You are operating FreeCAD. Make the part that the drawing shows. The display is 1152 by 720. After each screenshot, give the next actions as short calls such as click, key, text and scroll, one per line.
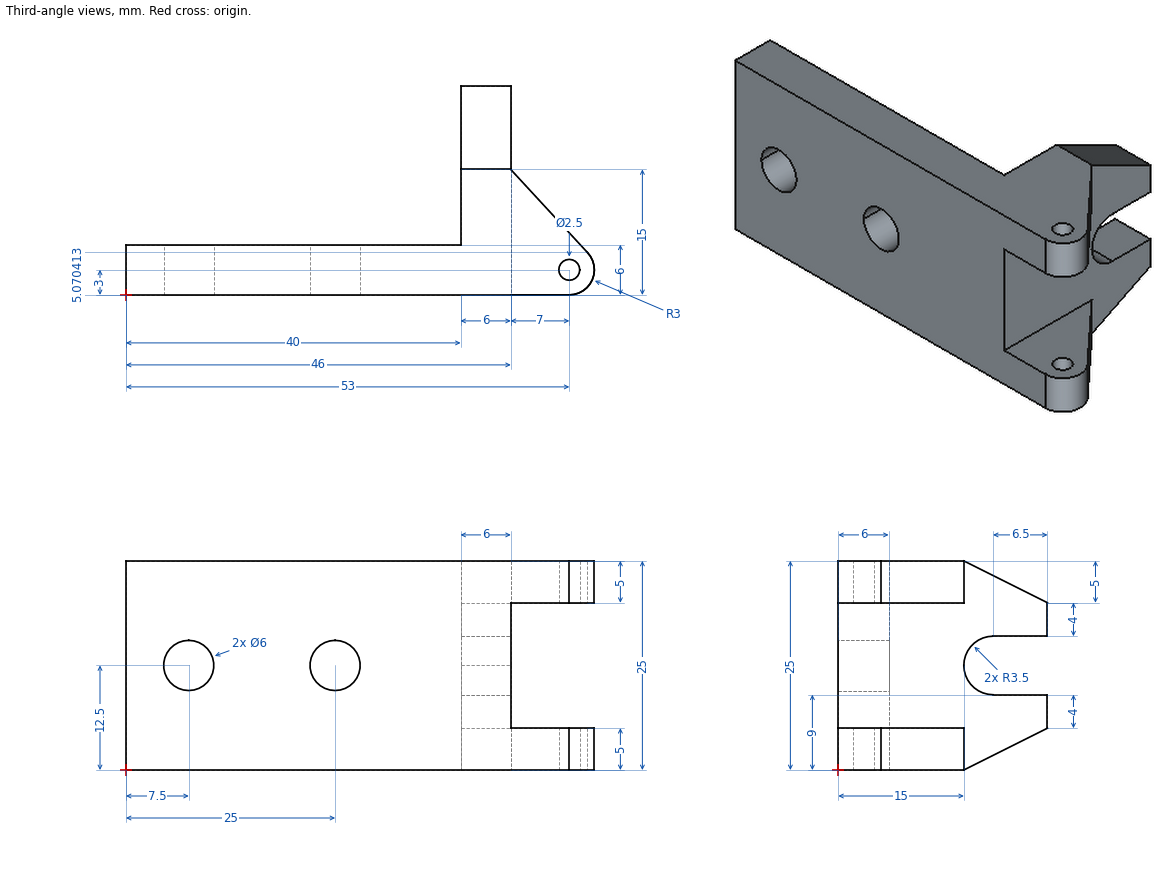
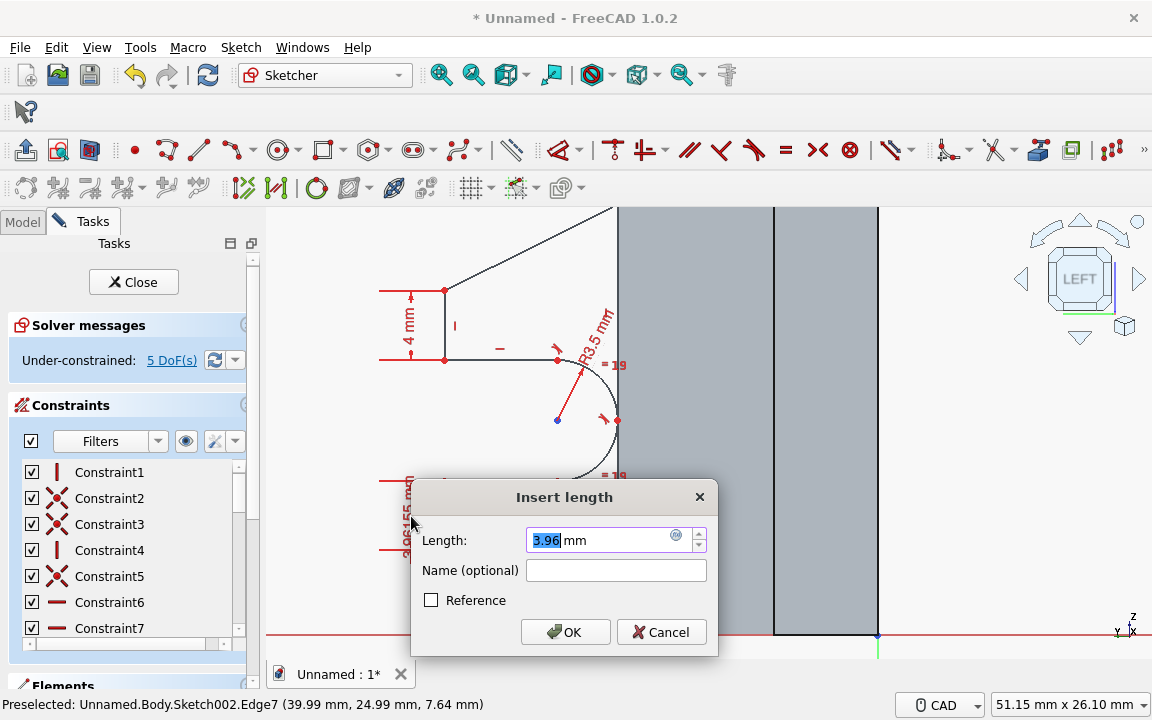
text(4)
key(Return)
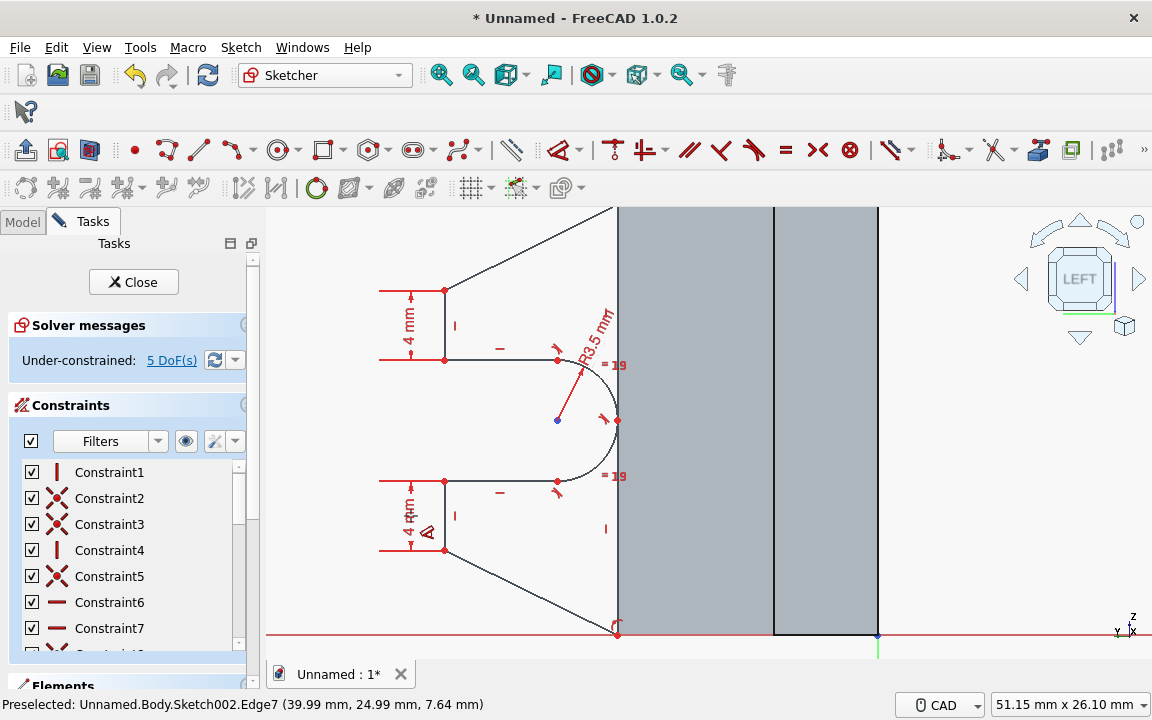
click(557, 481)
click(912, 556)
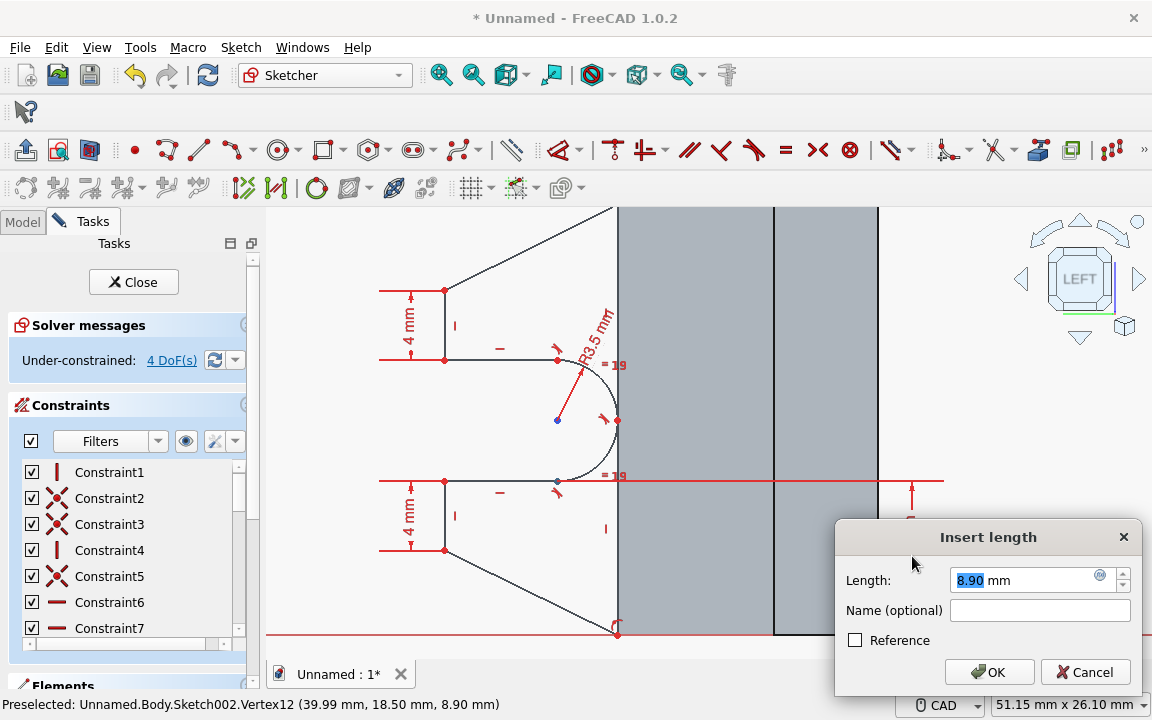
text(9)
key(Return)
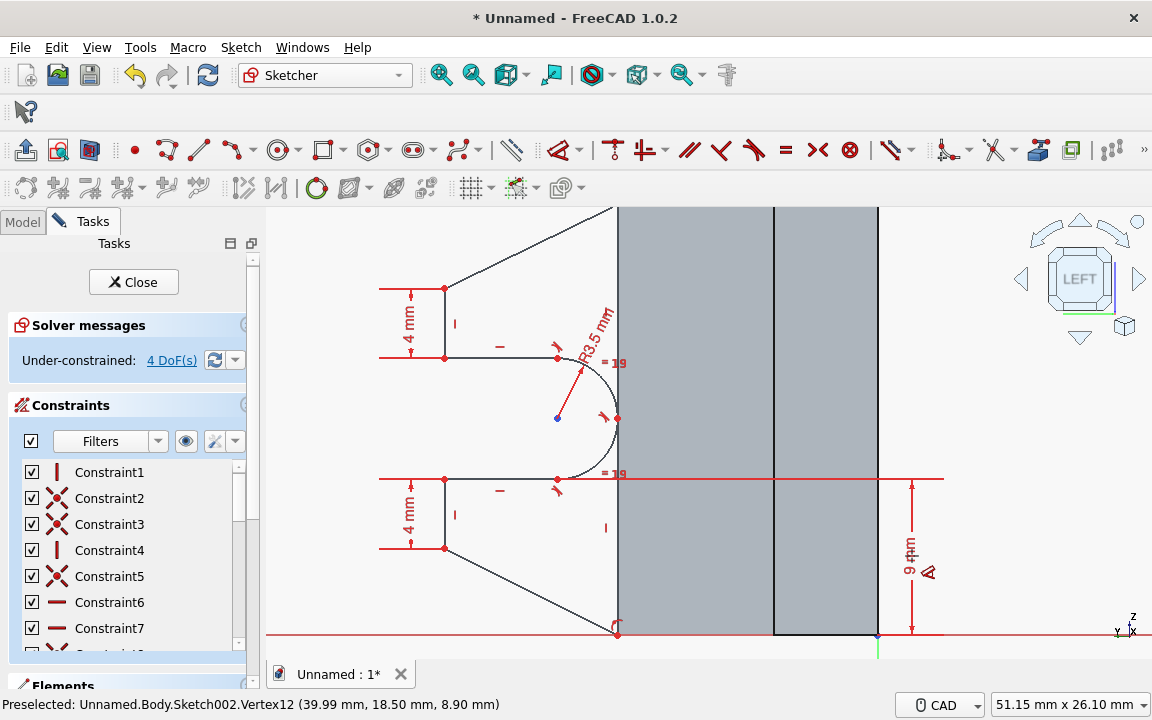
click(497, 264)
click(411, 262)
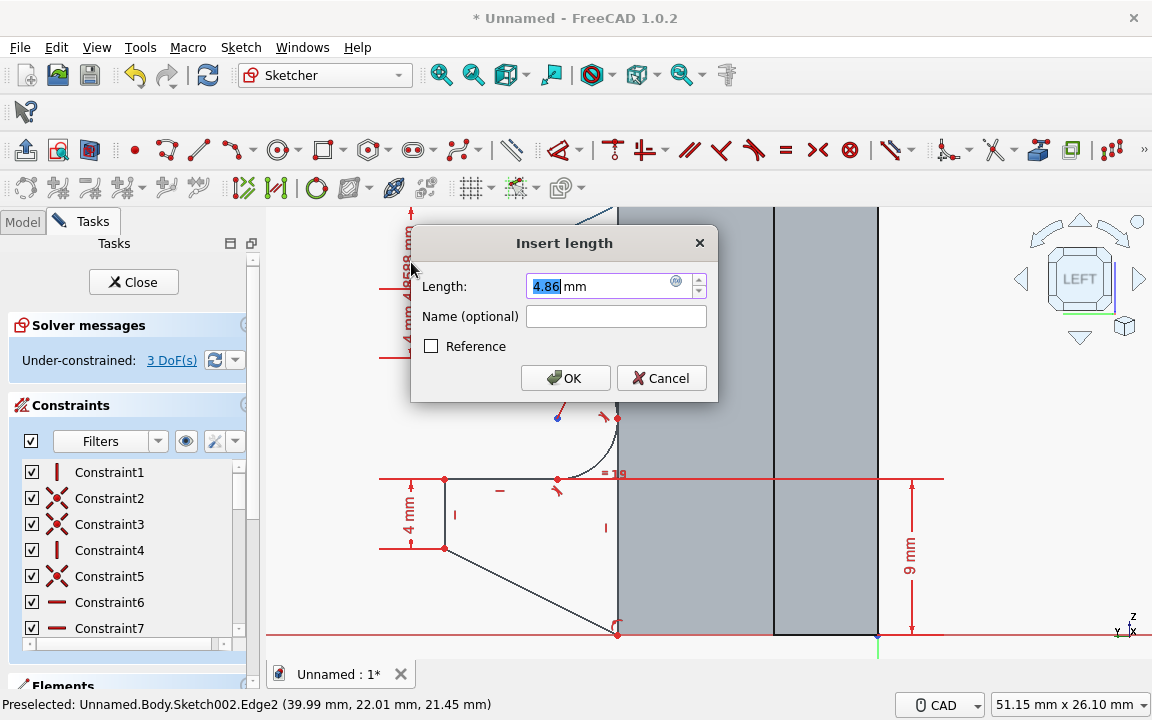
text(5)
key(Return)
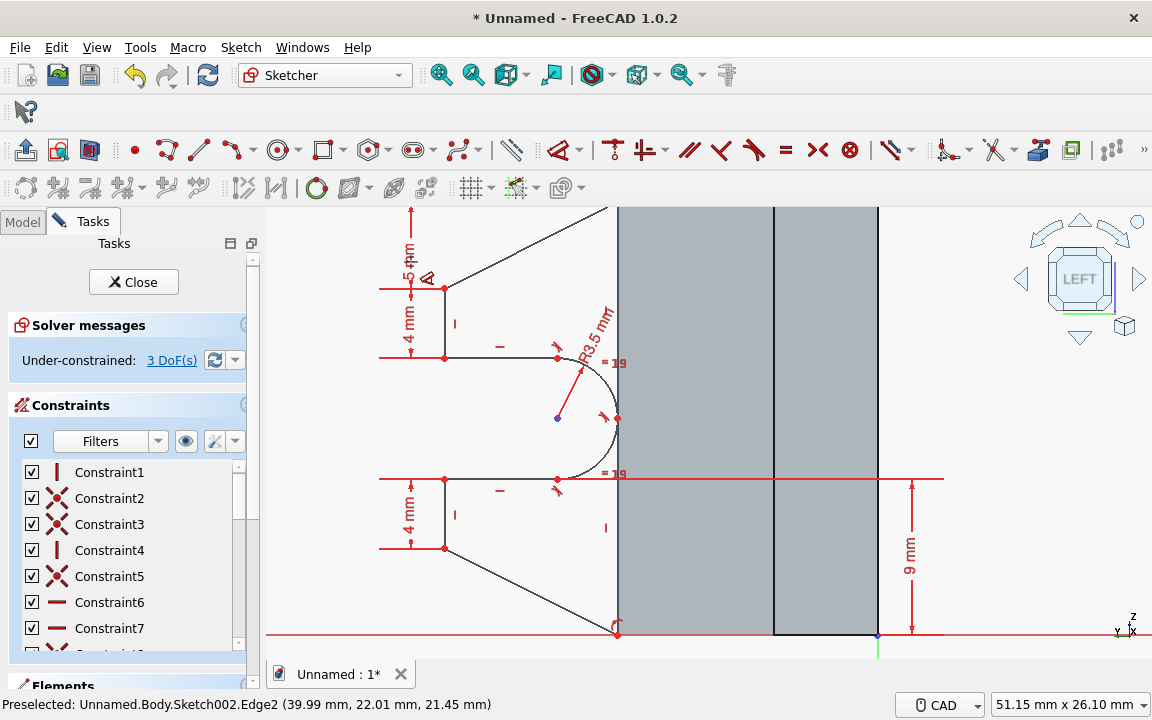
click(478, 358)
click(501, 324)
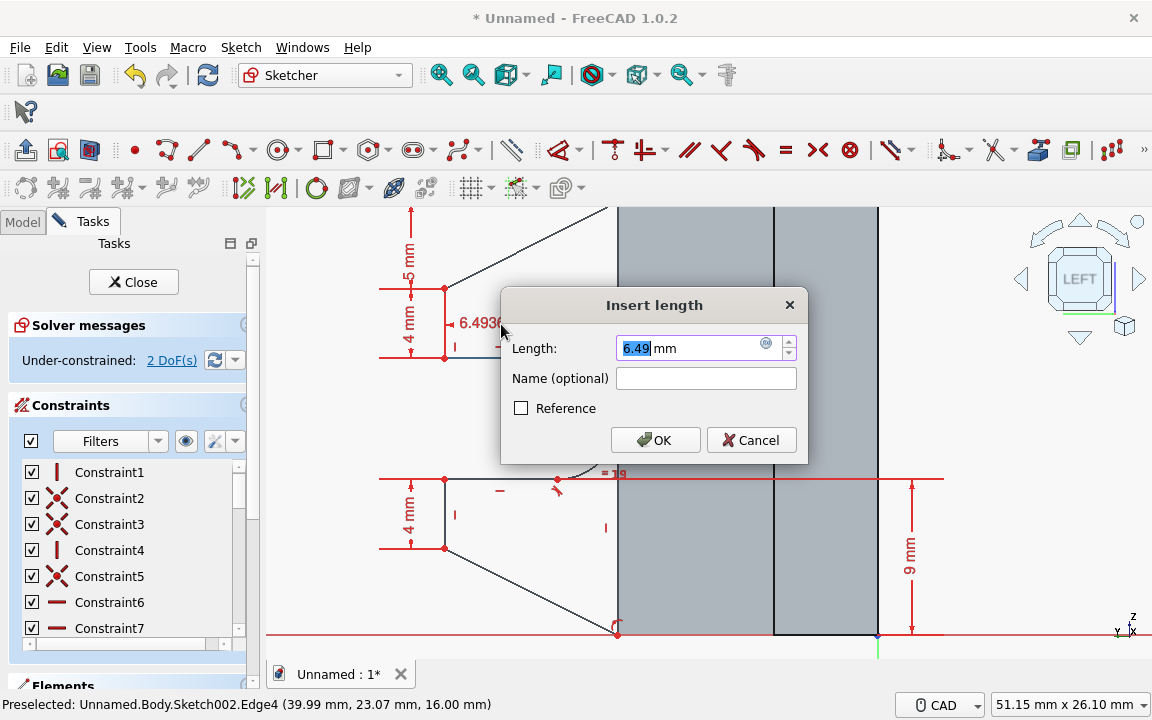
text(6.5)
key(Return)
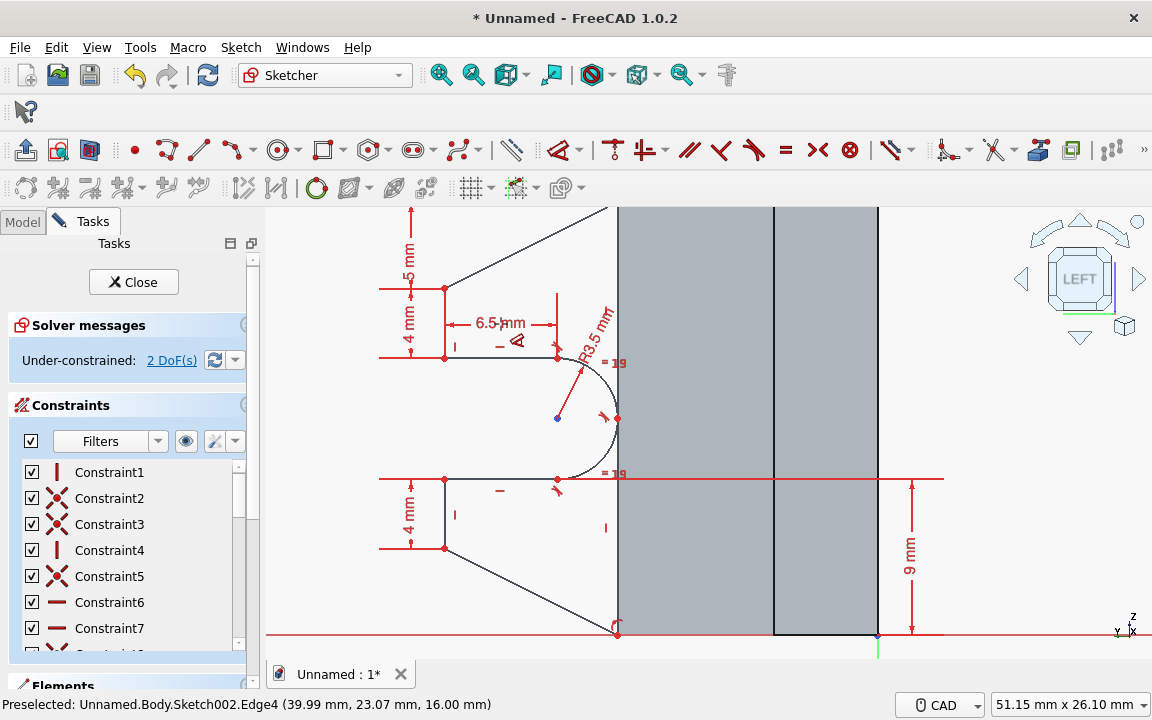
click(523, 479)
click(501, 513)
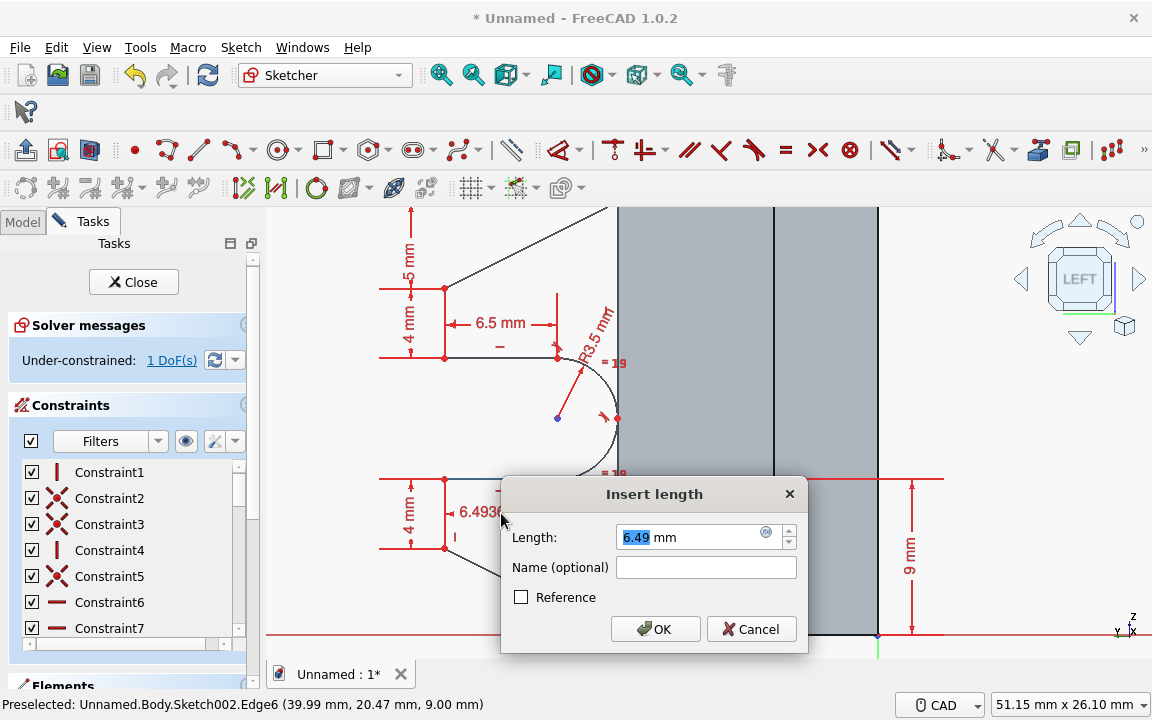
text(6.5)
key(Return)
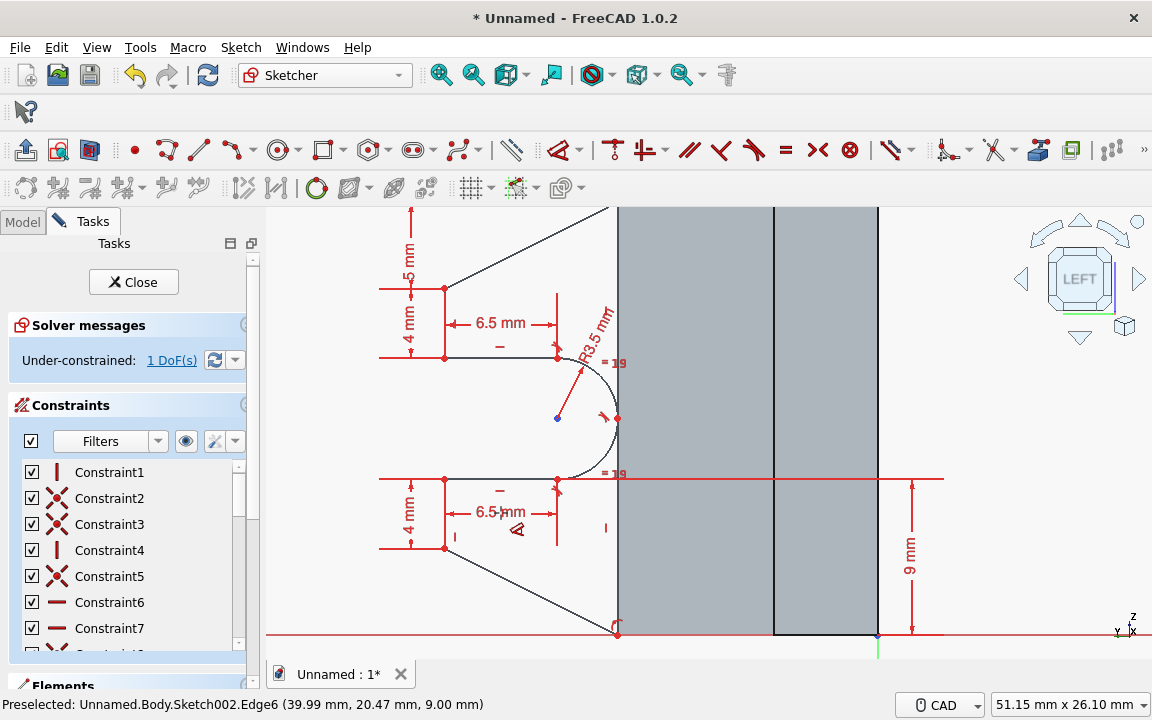
click(618, 419)
click(748, 385)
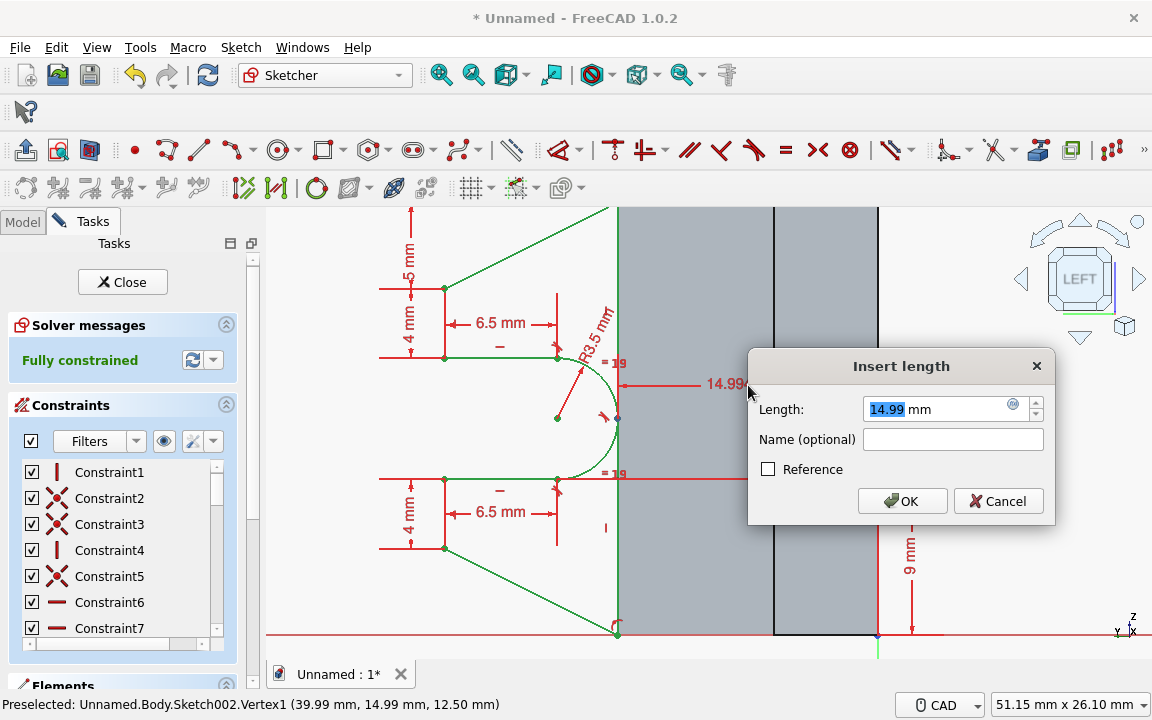
text(15)
key(Return)
key(Escape)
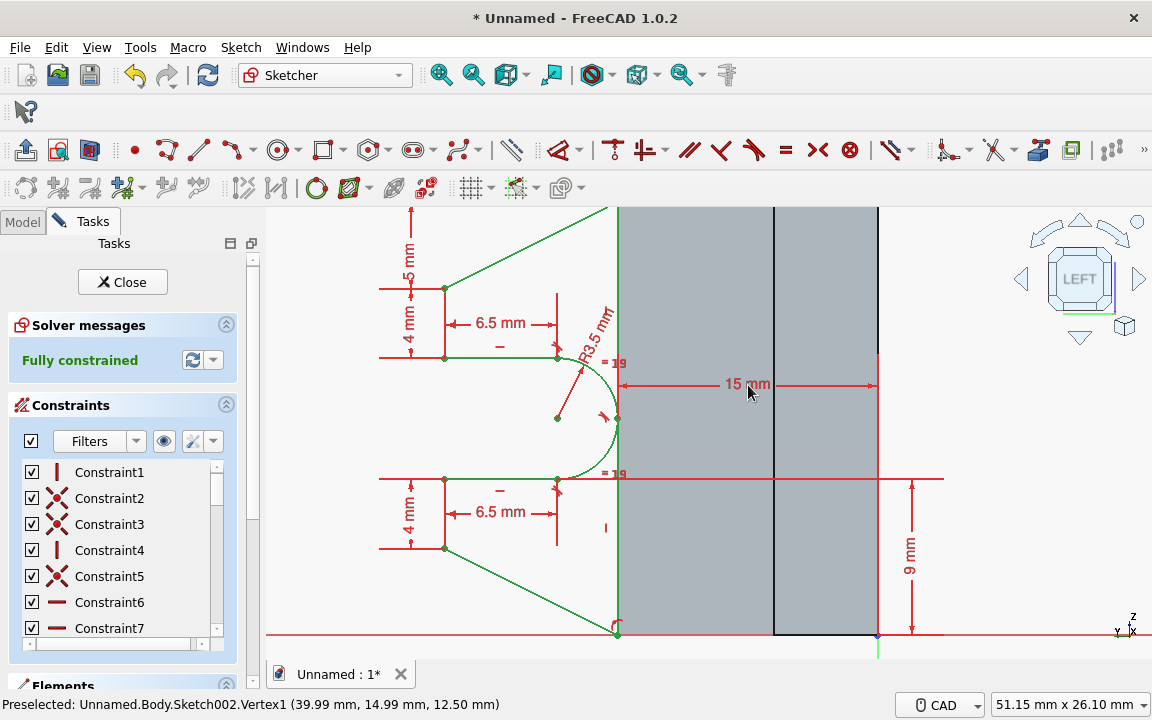
click(123, 282)